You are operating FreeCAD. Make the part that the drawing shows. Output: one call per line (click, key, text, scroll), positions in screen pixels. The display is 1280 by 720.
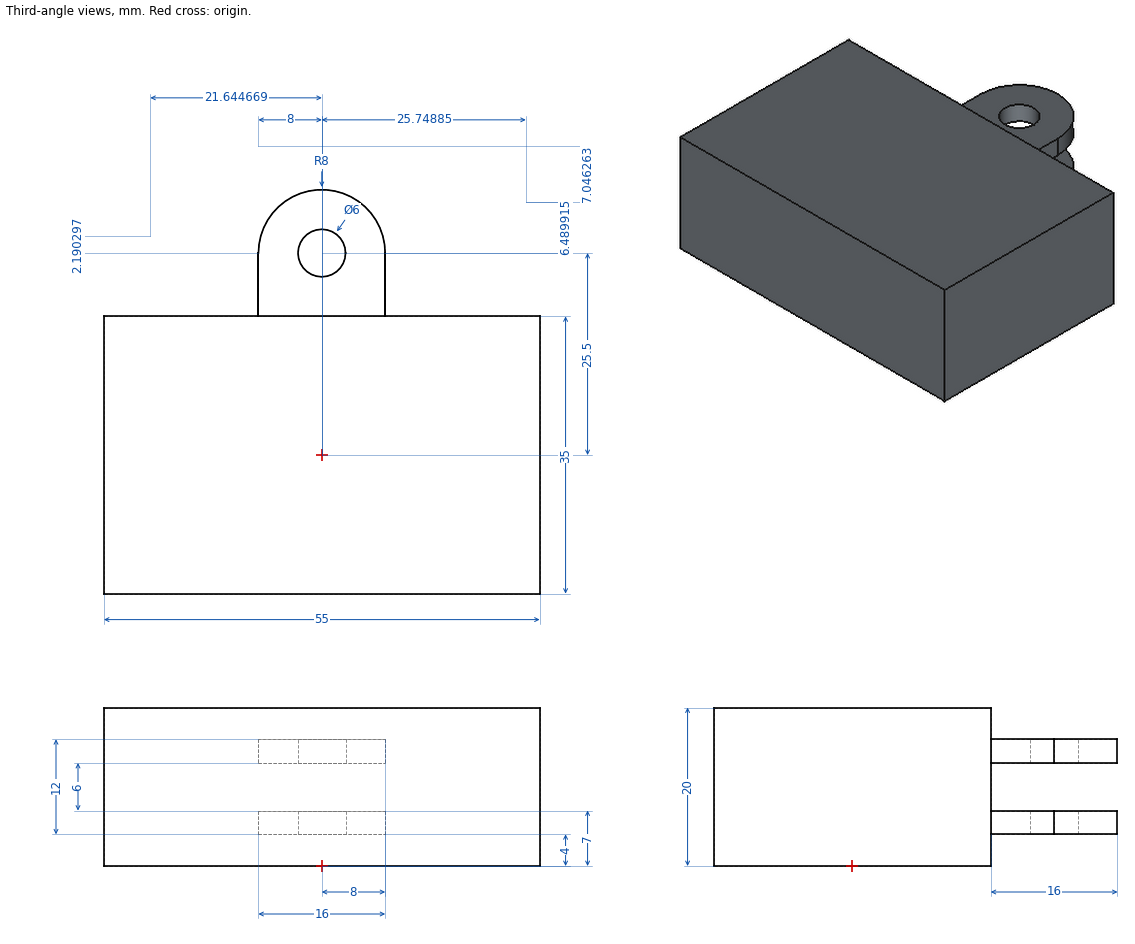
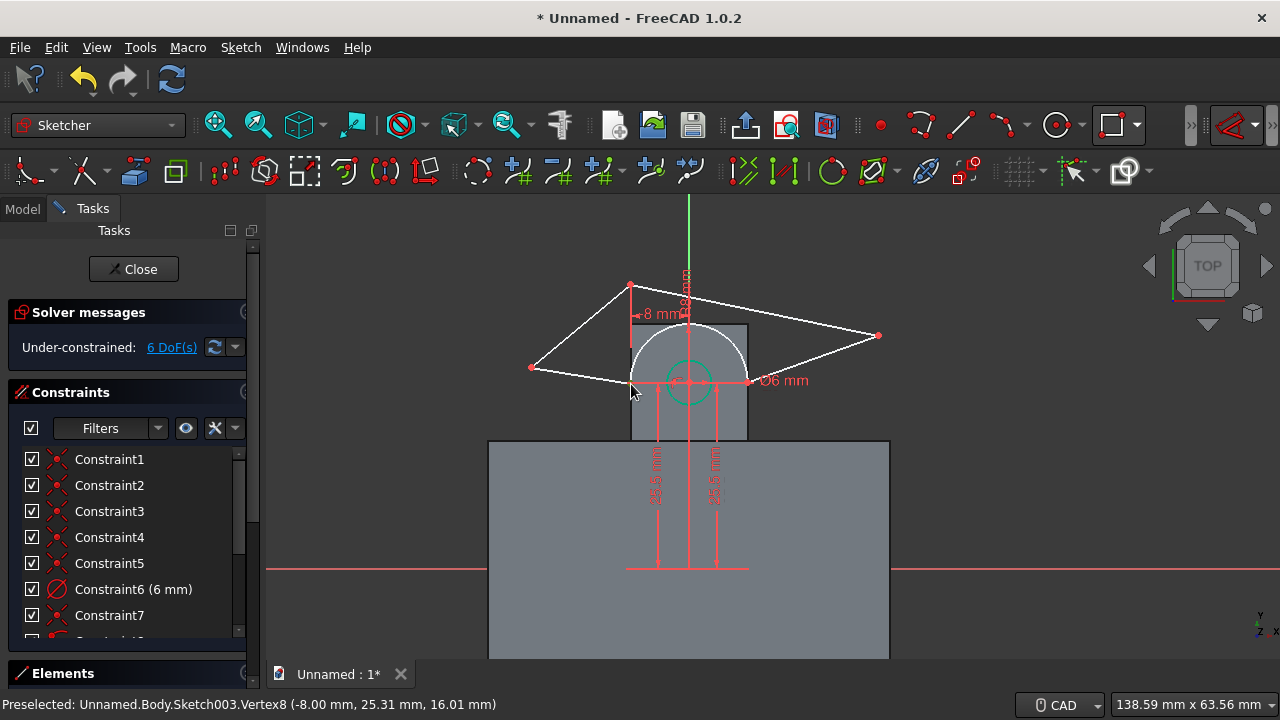
click(1258, 126)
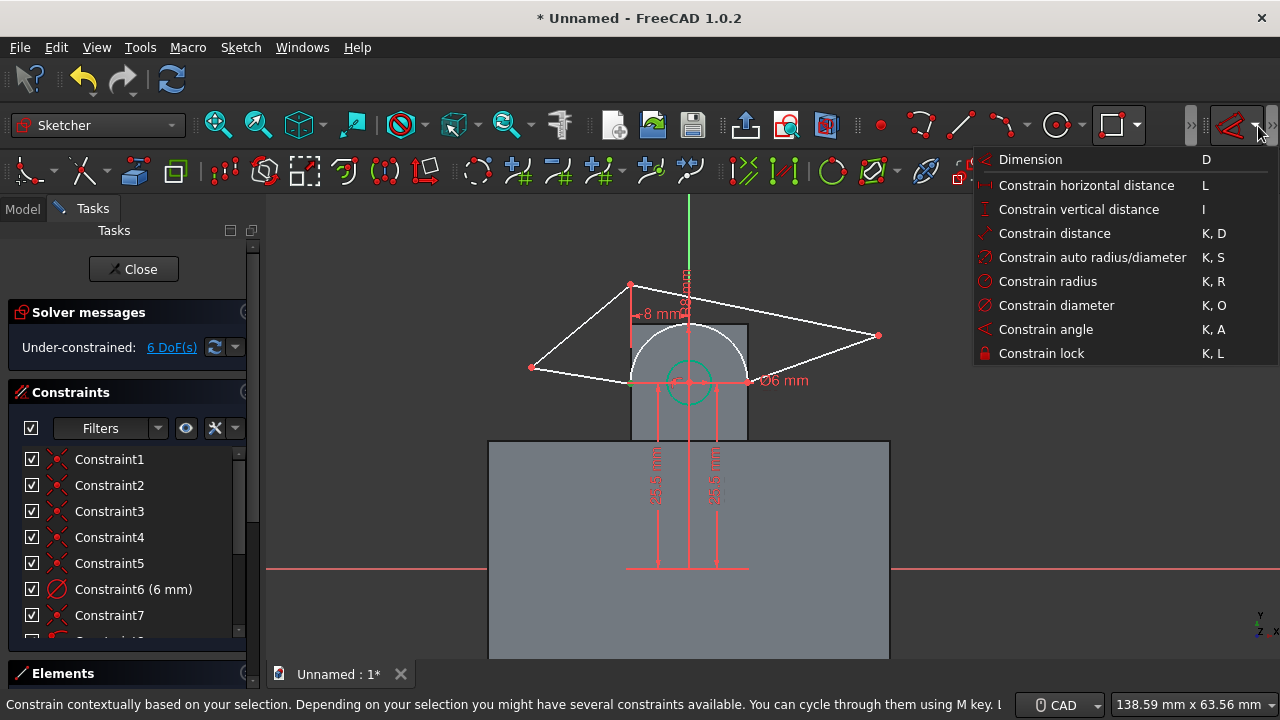
click(1126, 209)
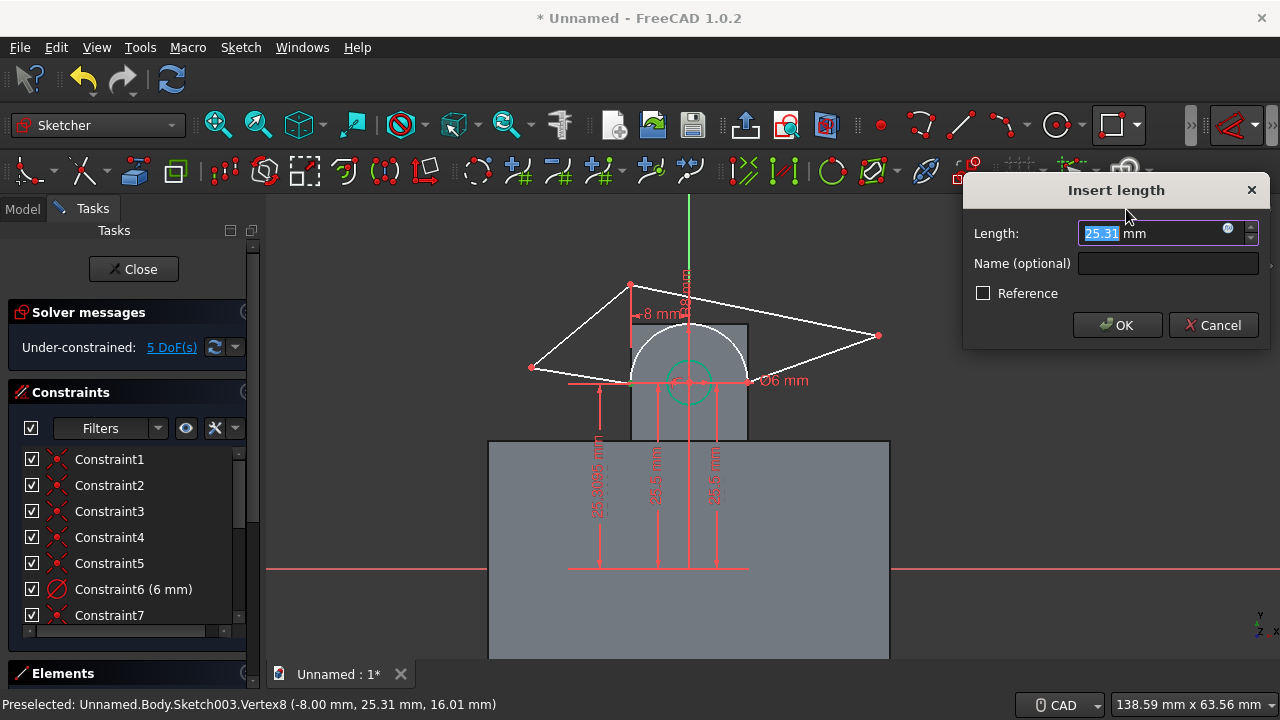
text(25.5)
key(Return)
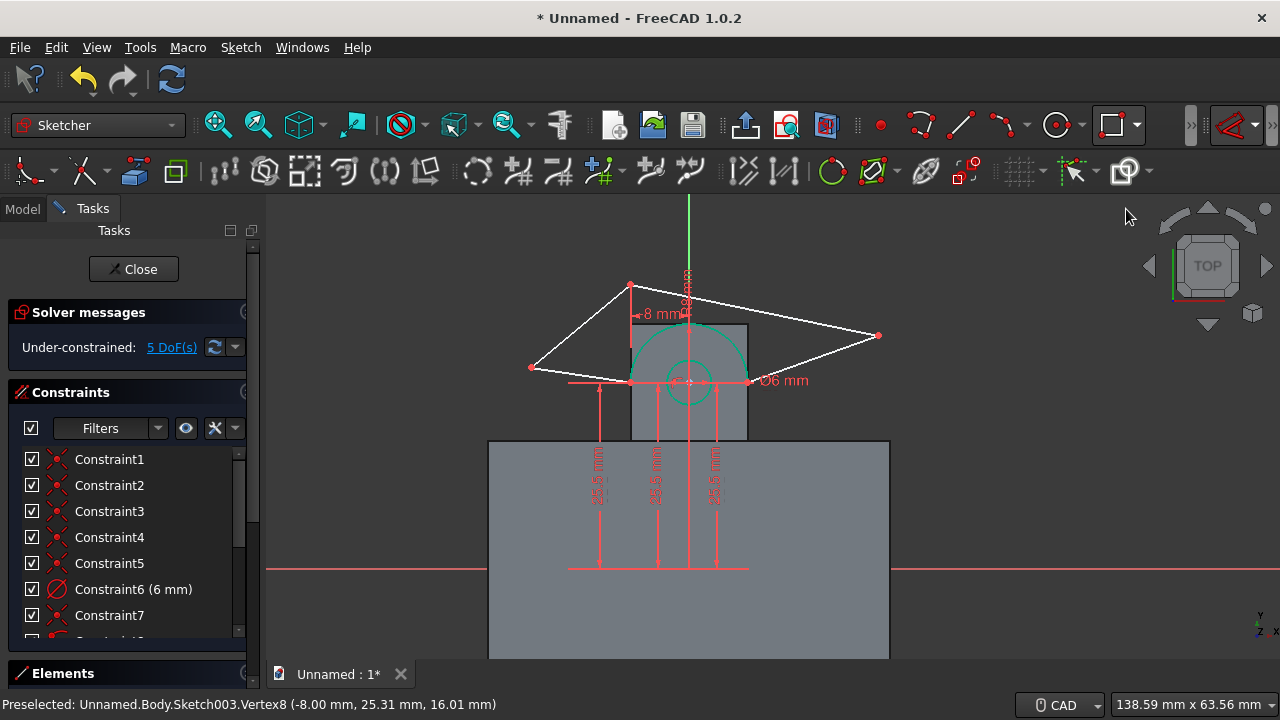
click(878, 336)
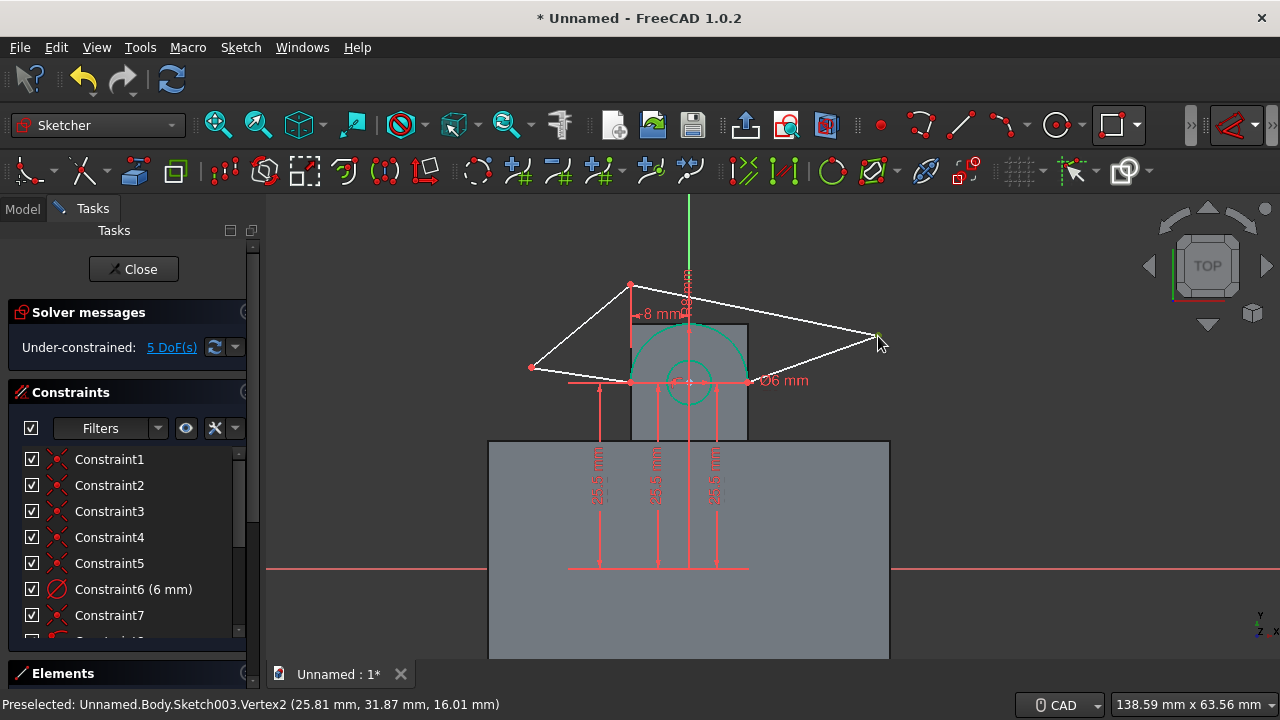
click(1258, 126)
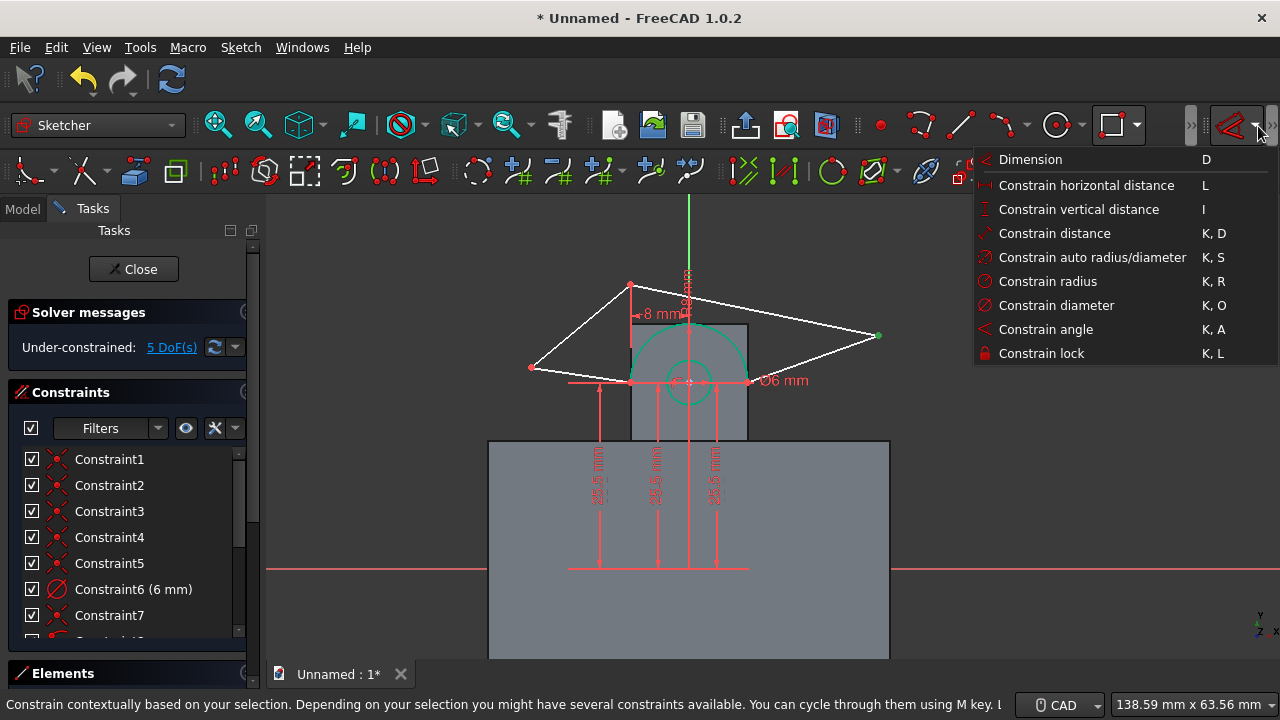
click(1126, 185)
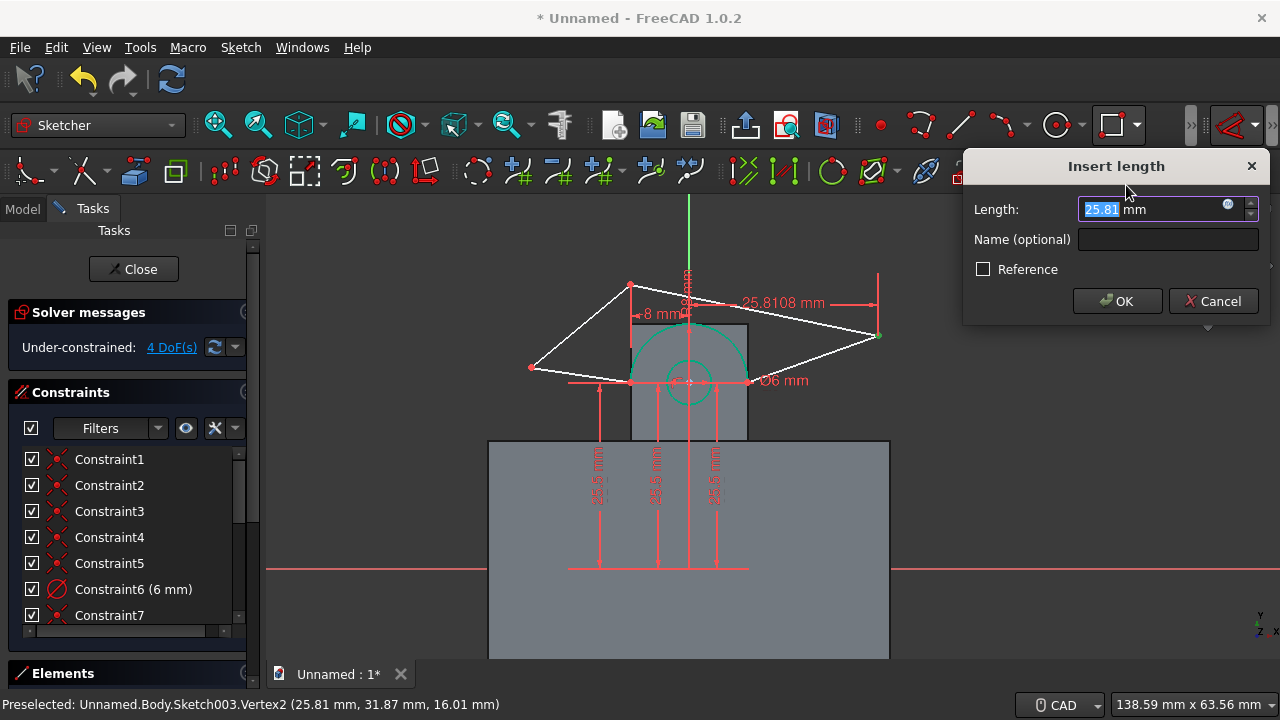
text(25.74885)
key(Return)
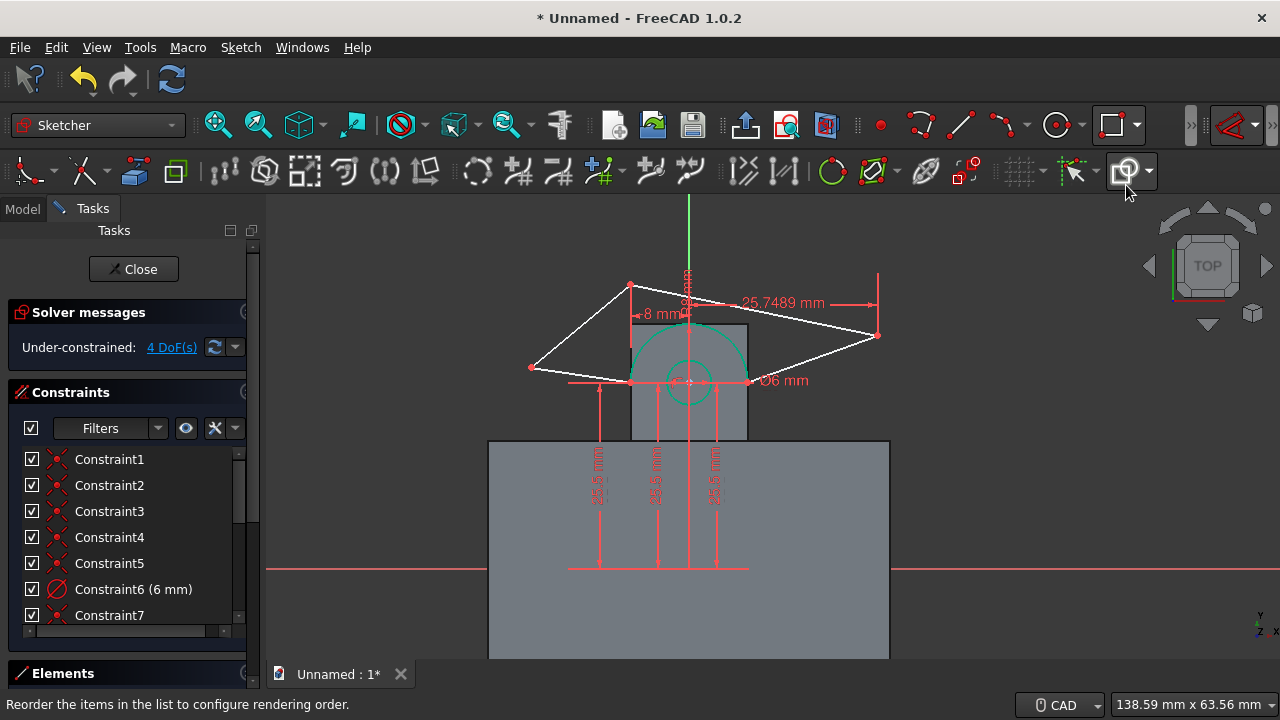
click(787, 369)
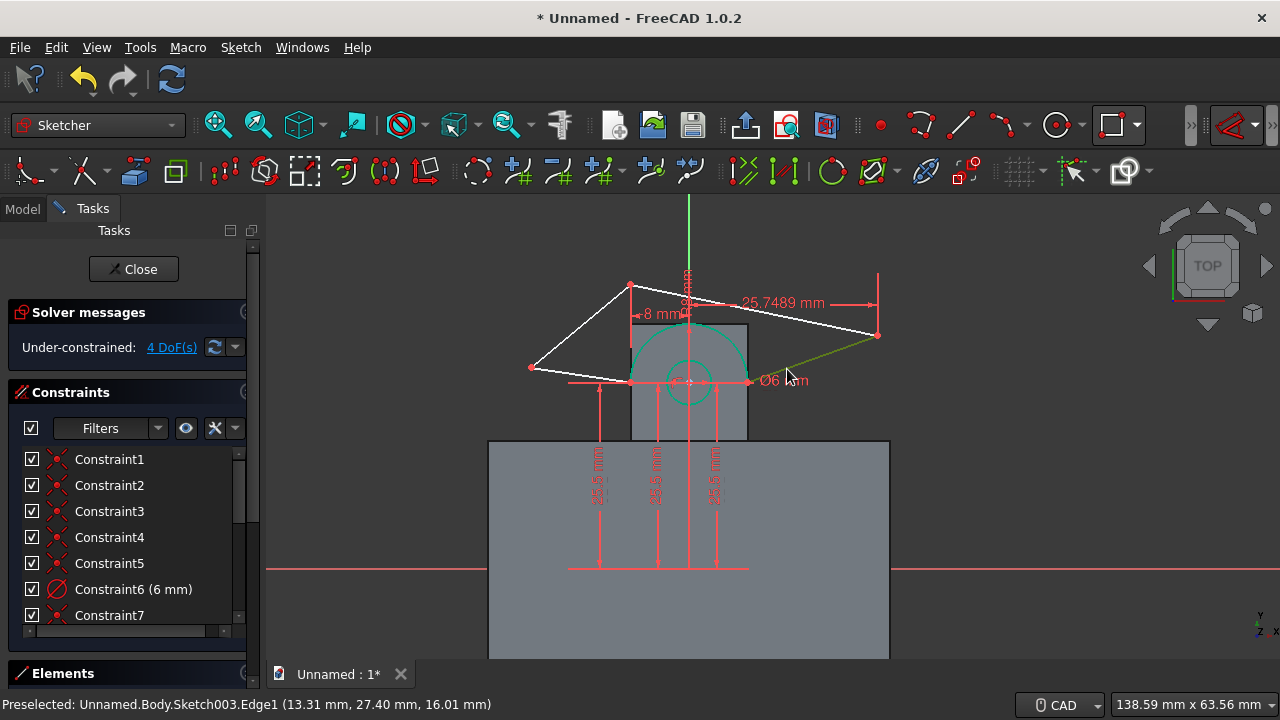
key(i)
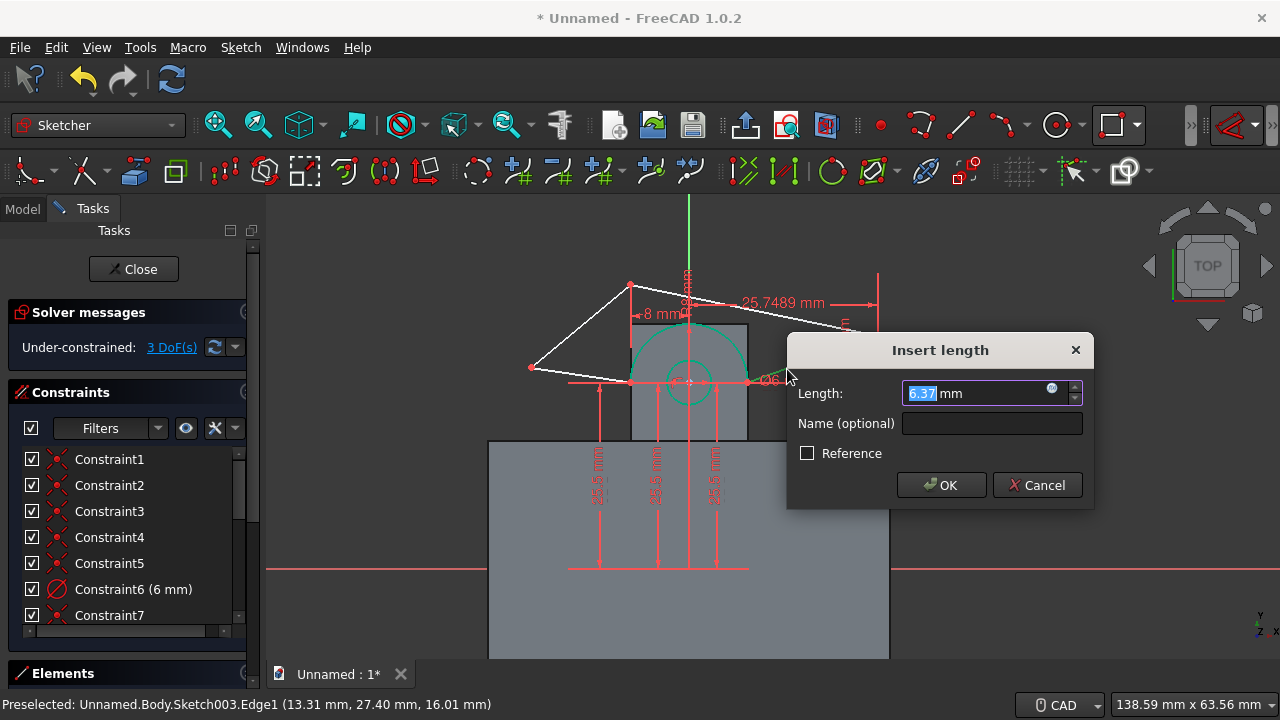
text(6.489915)
key(Return)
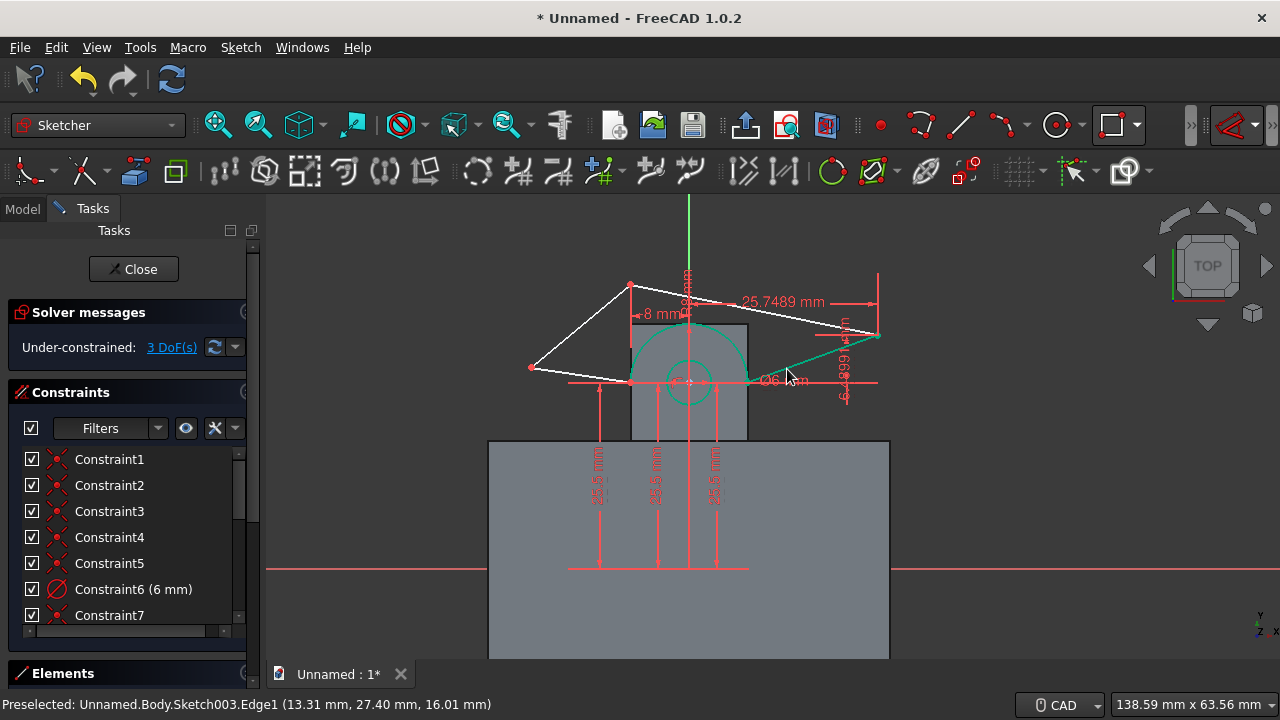
click(803, 320)